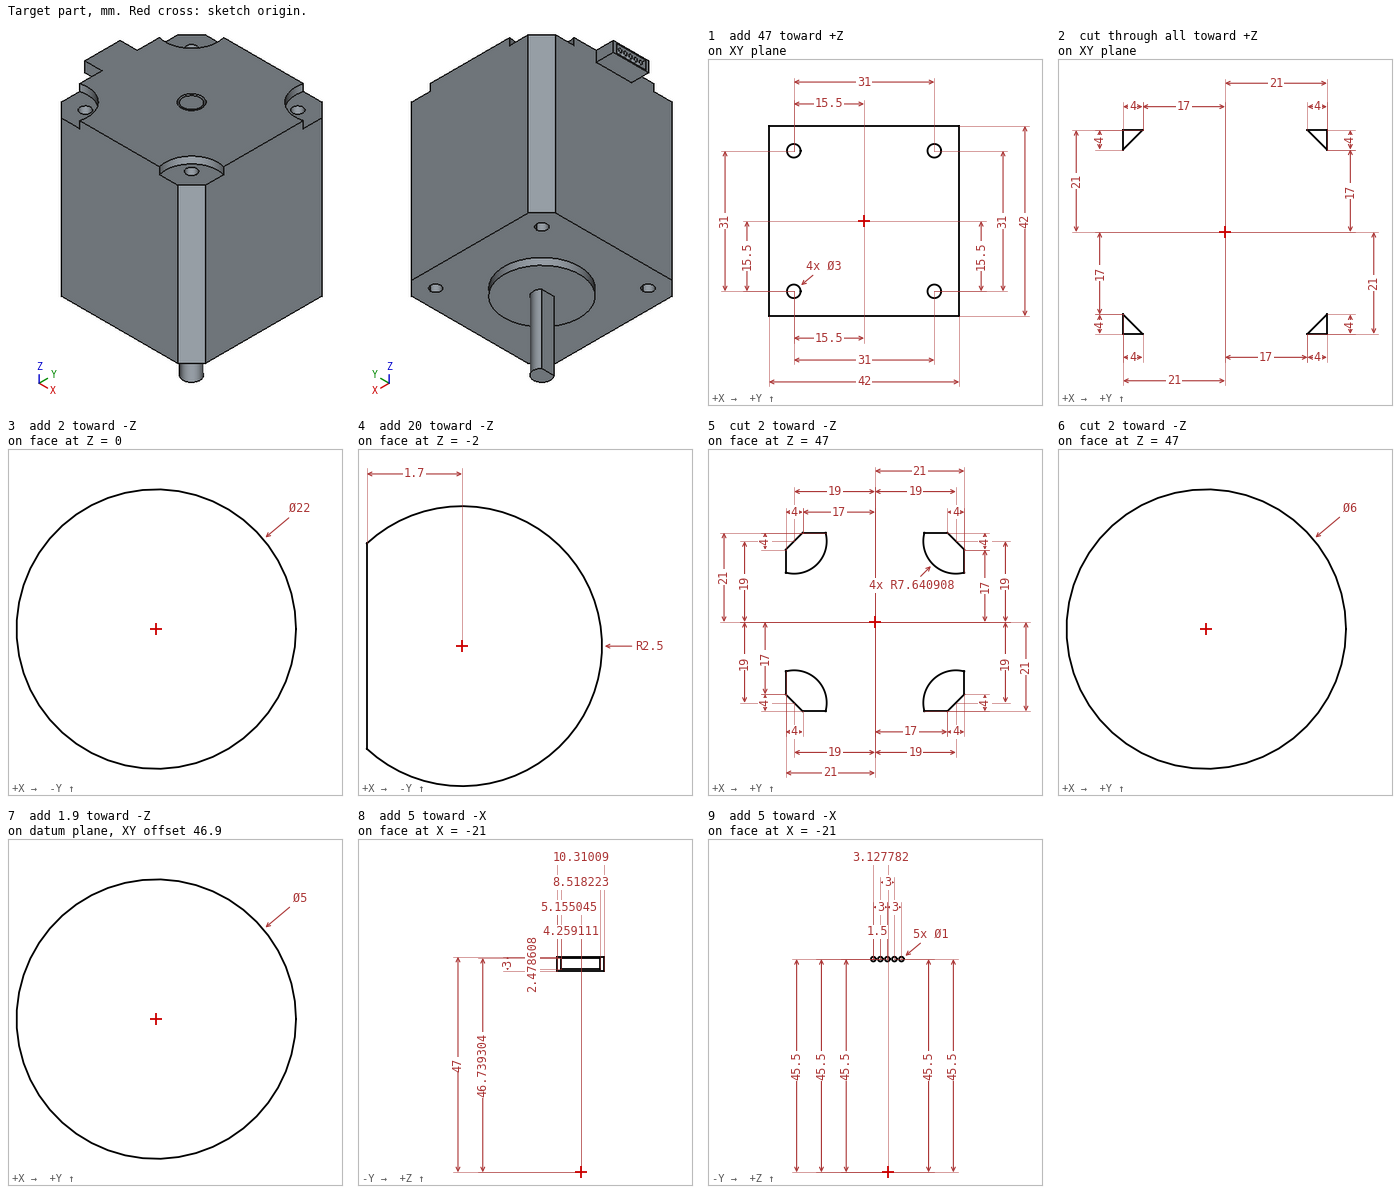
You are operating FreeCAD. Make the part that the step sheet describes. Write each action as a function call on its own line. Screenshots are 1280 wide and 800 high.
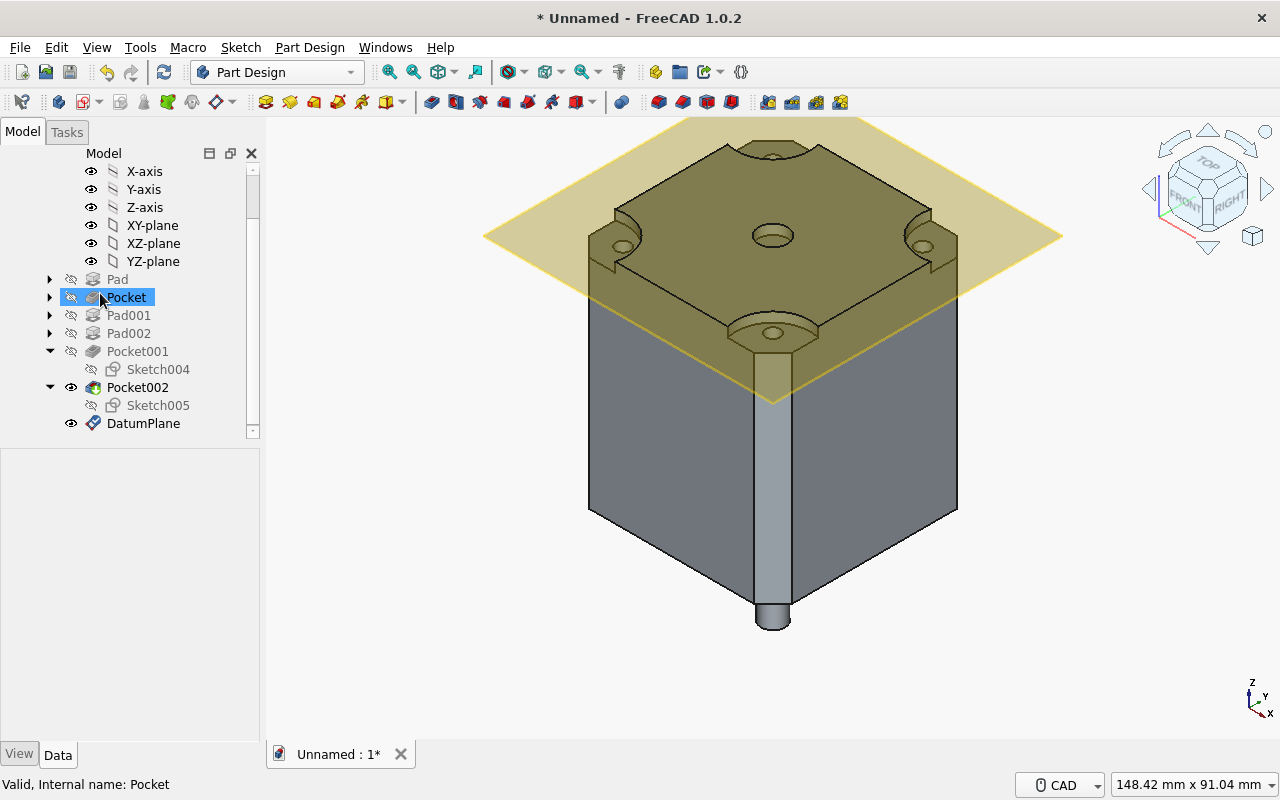
click(116, 423)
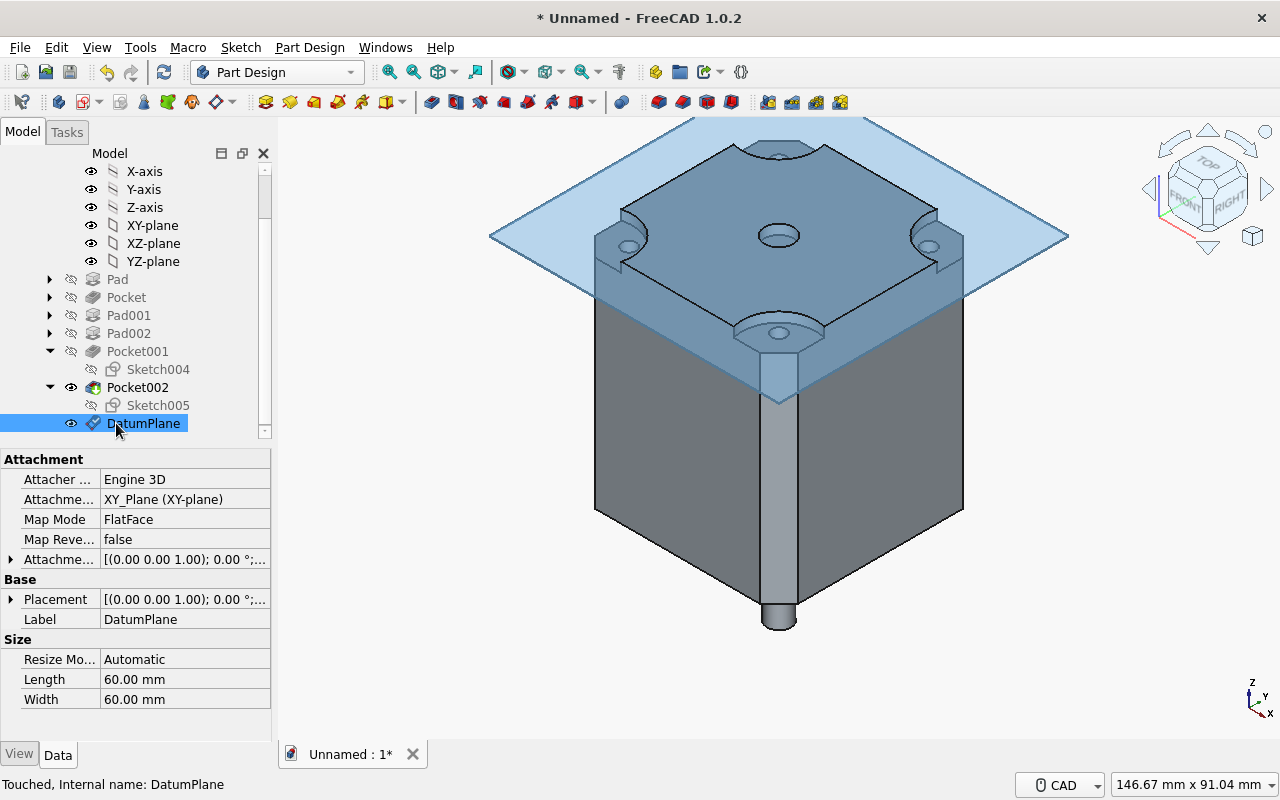
click(84, 102)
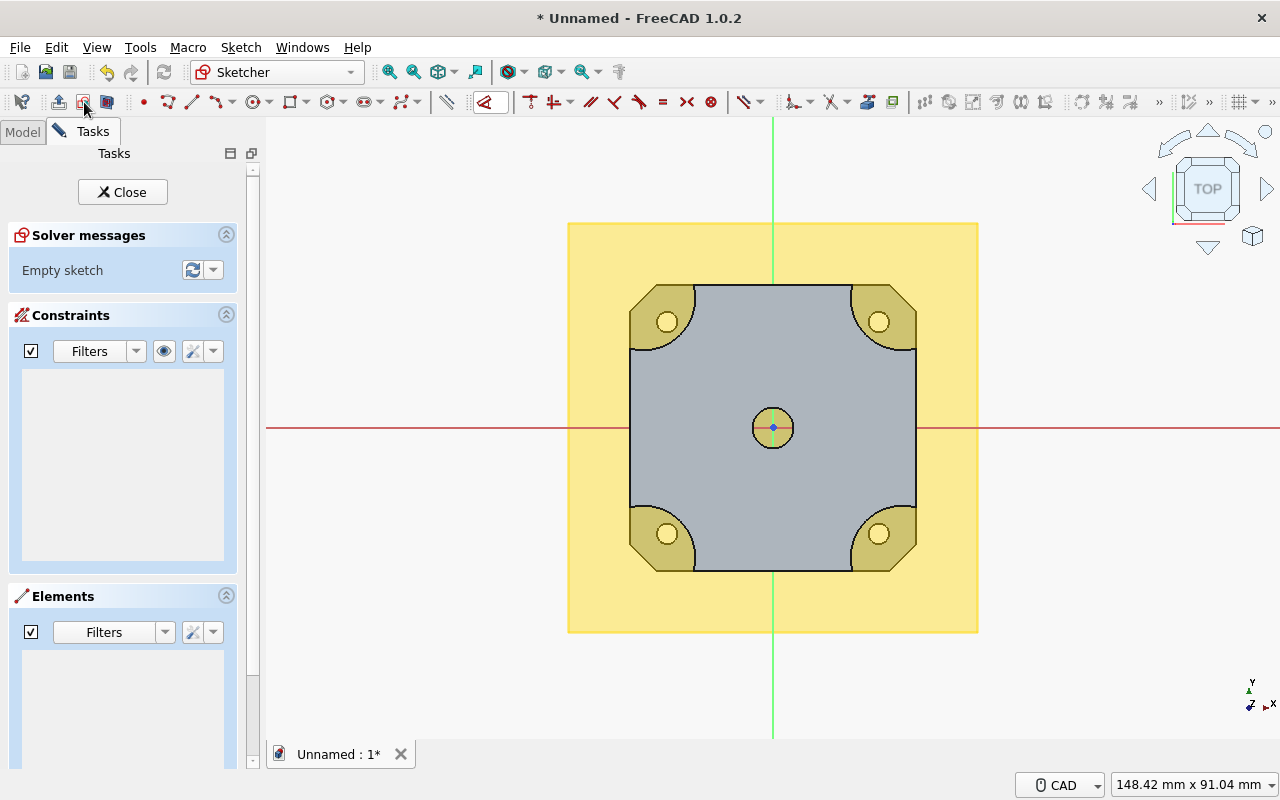
click(108, 102)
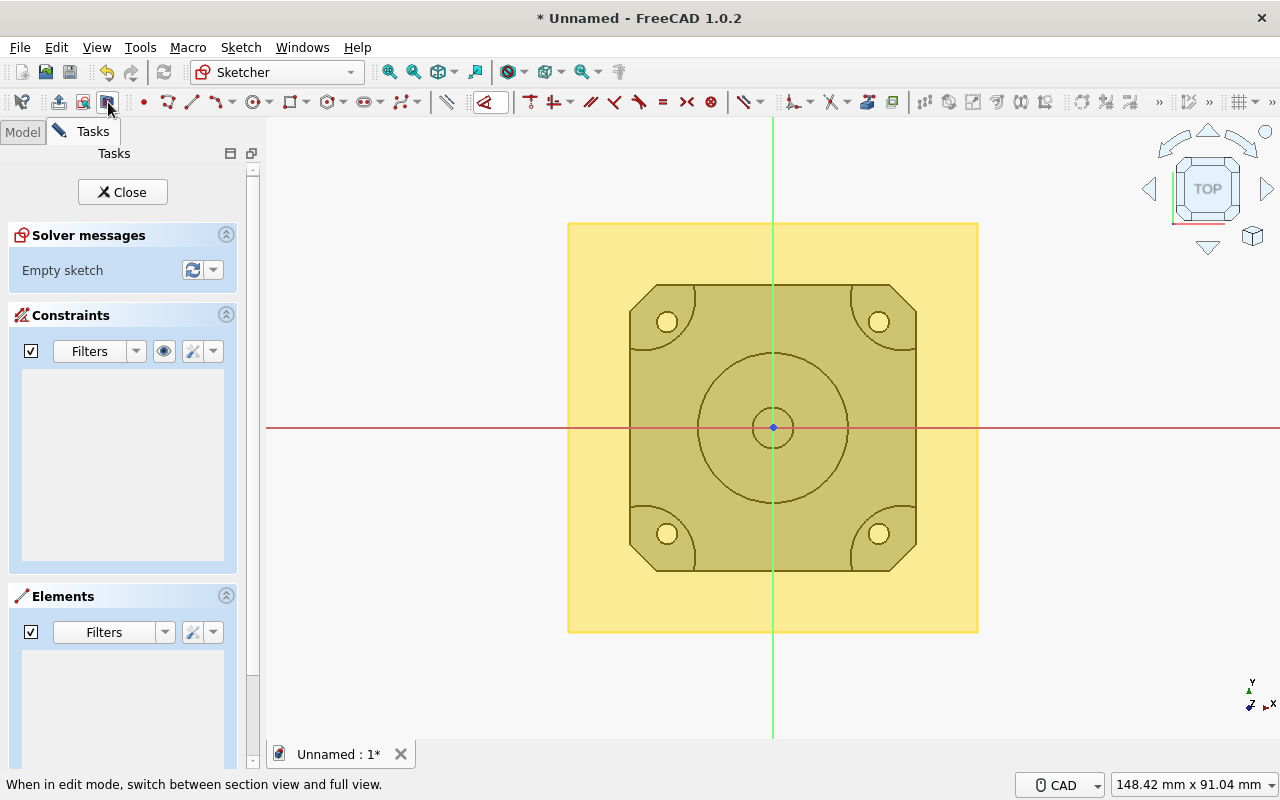
scroll(780, 428, up, 12)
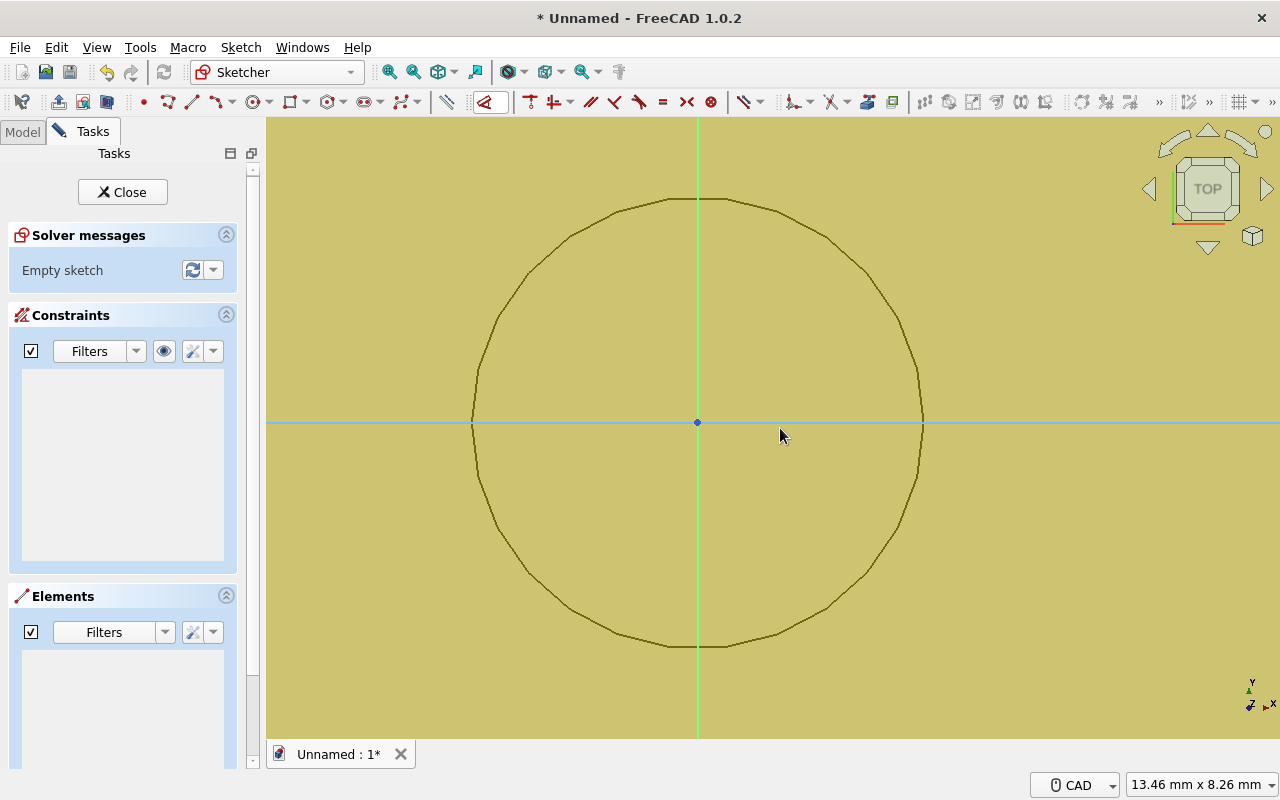
click(254, 102)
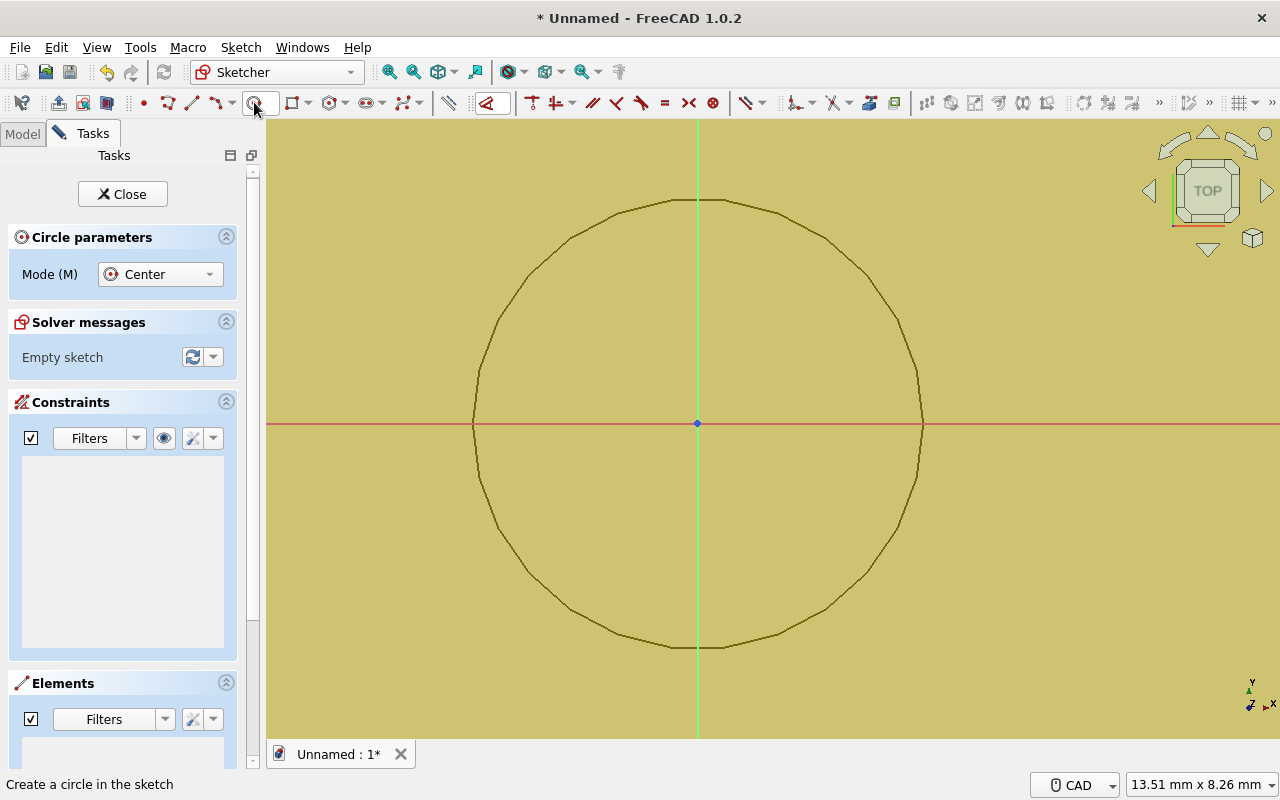
click(698, 424)
click(831, 291)
key(Escape)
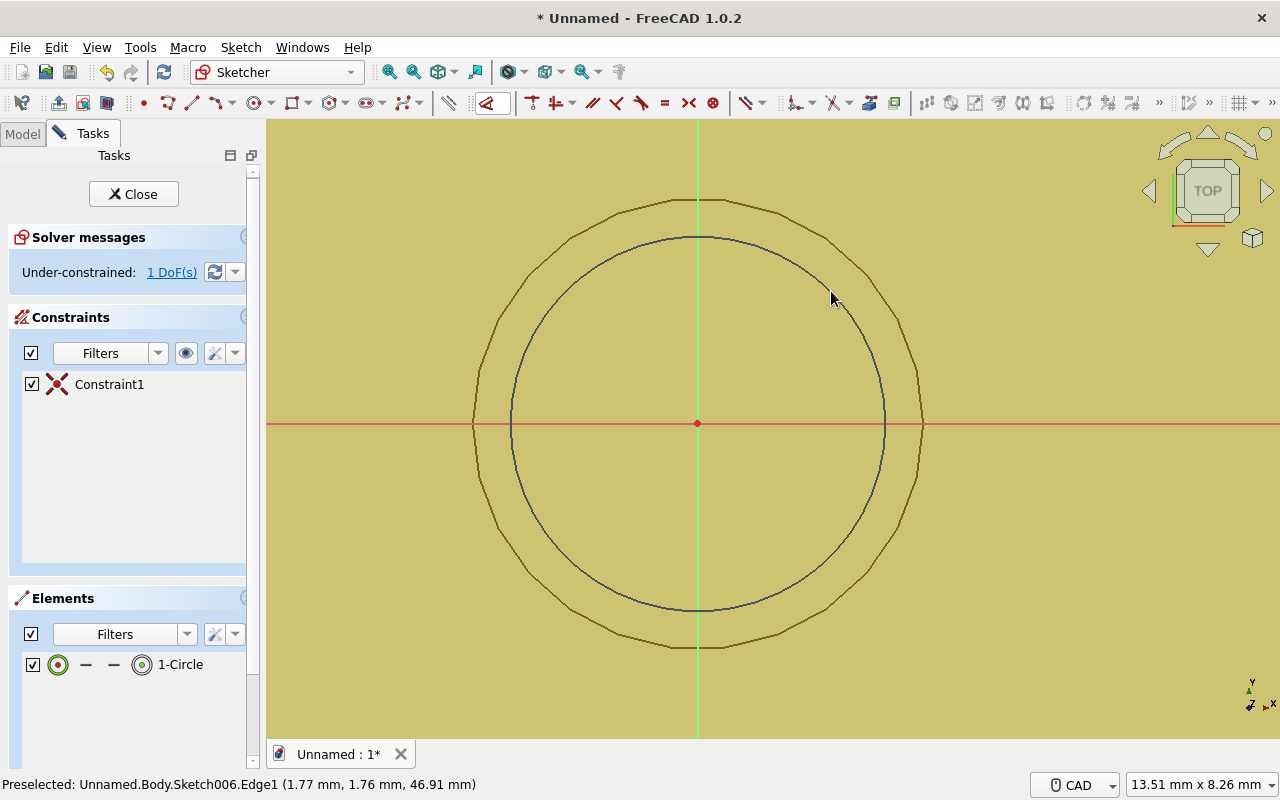
click(830, 291)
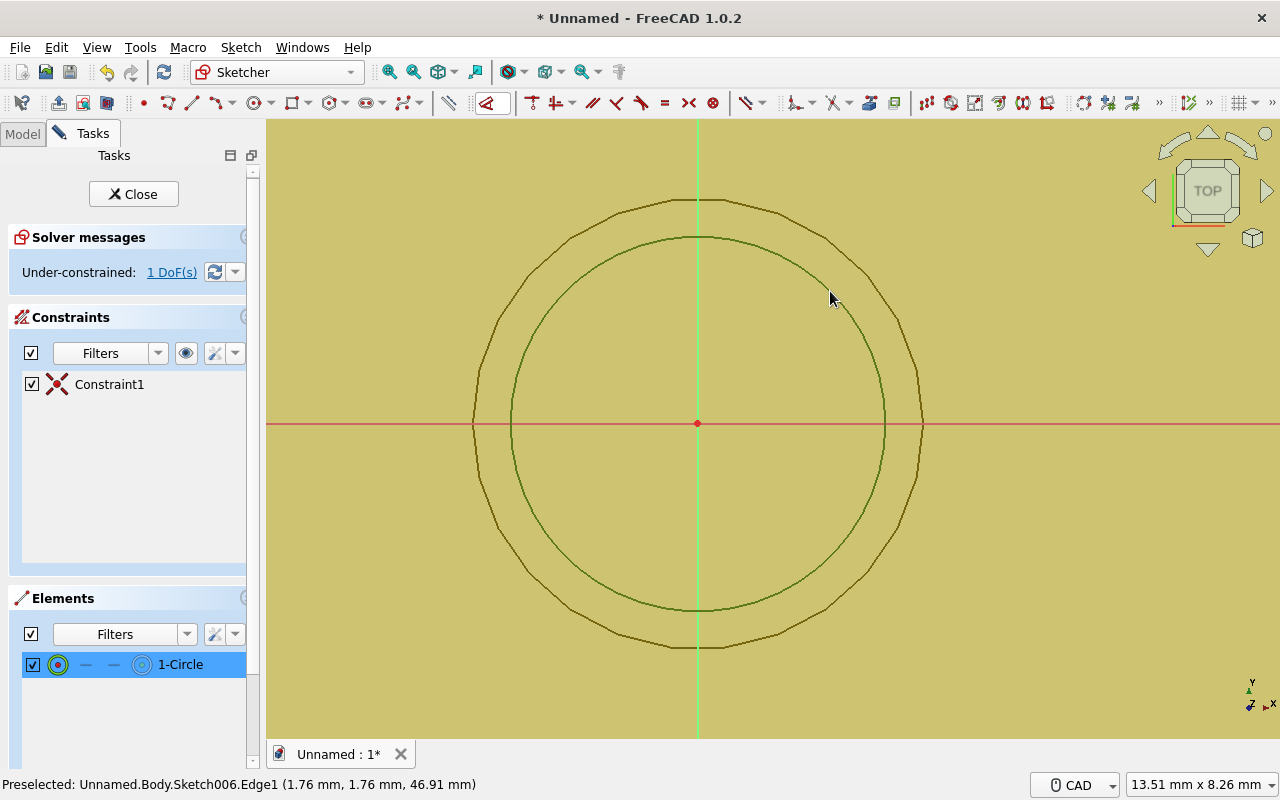
key(k)
key(o)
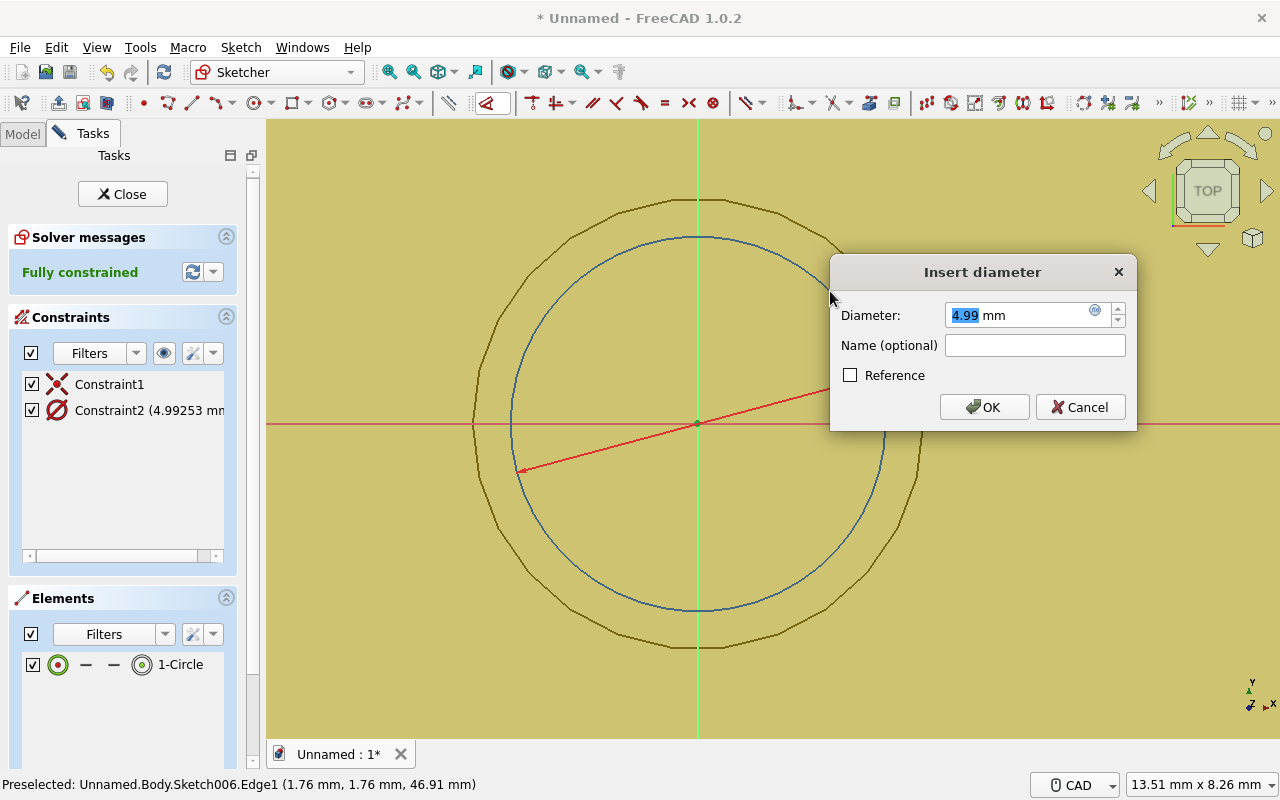
text(5)
key(Return)